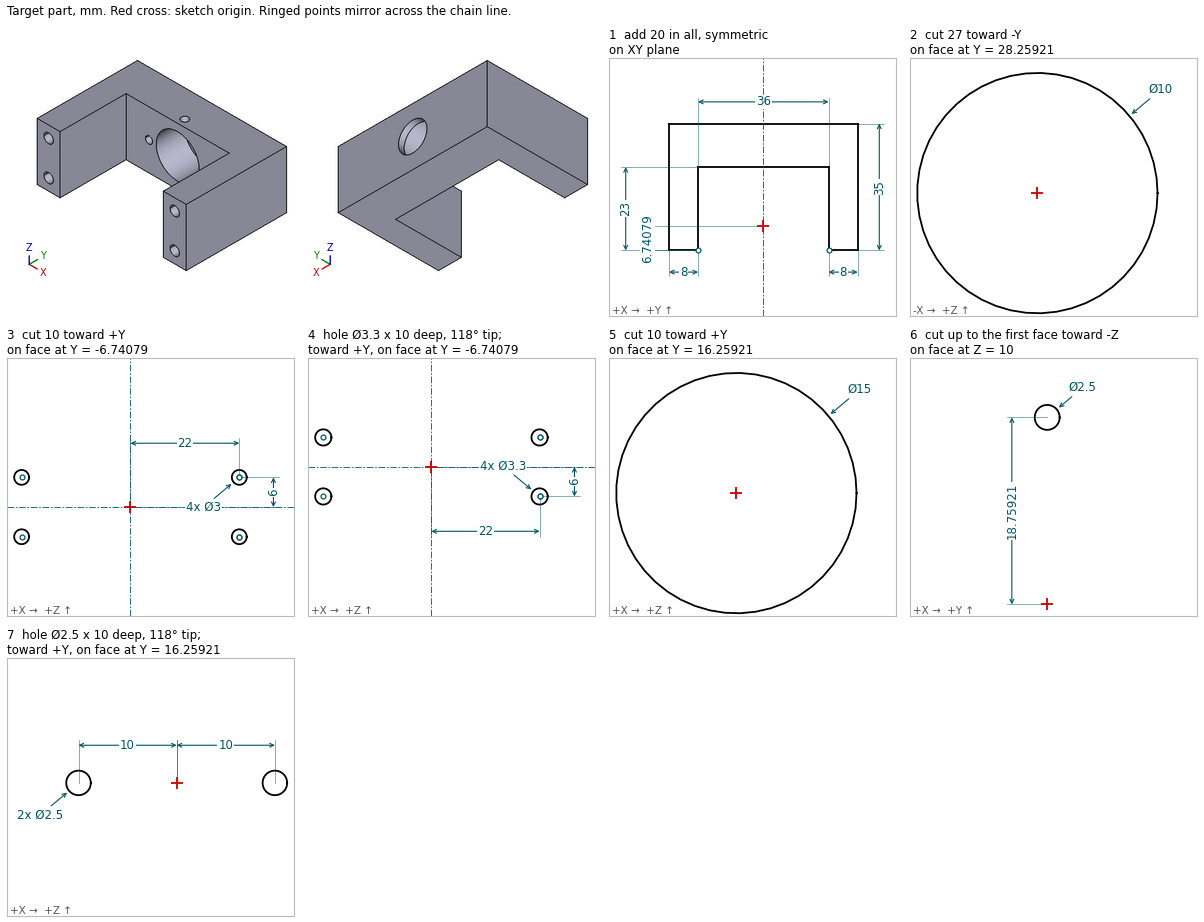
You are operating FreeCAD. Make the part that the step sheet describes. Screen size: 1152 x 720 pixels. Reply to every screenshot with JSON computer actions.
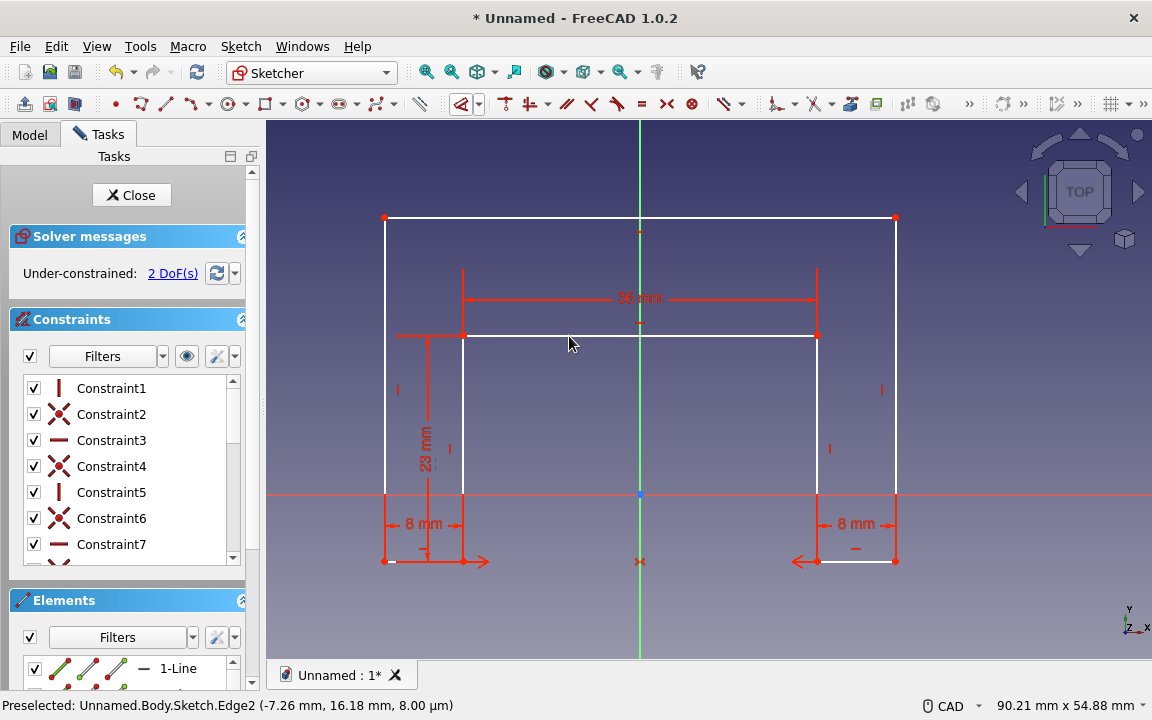
{"action": "left_click", "coordinate": [896, 459]}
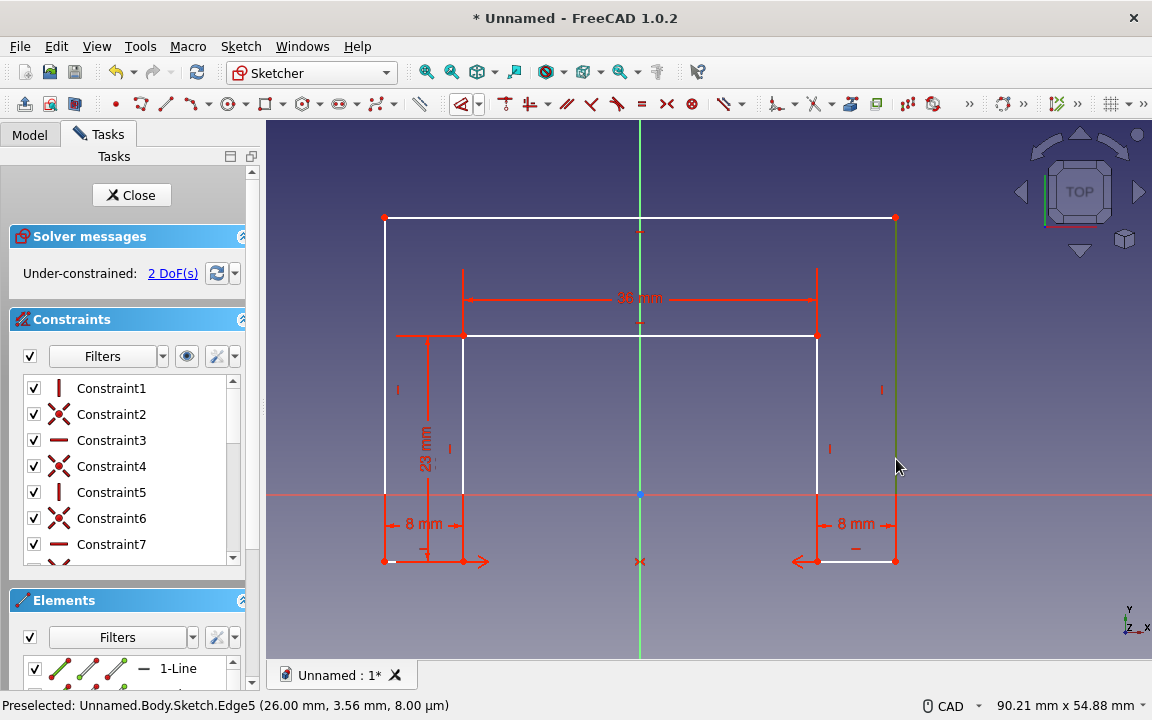
{"action": "key", "text": "i"}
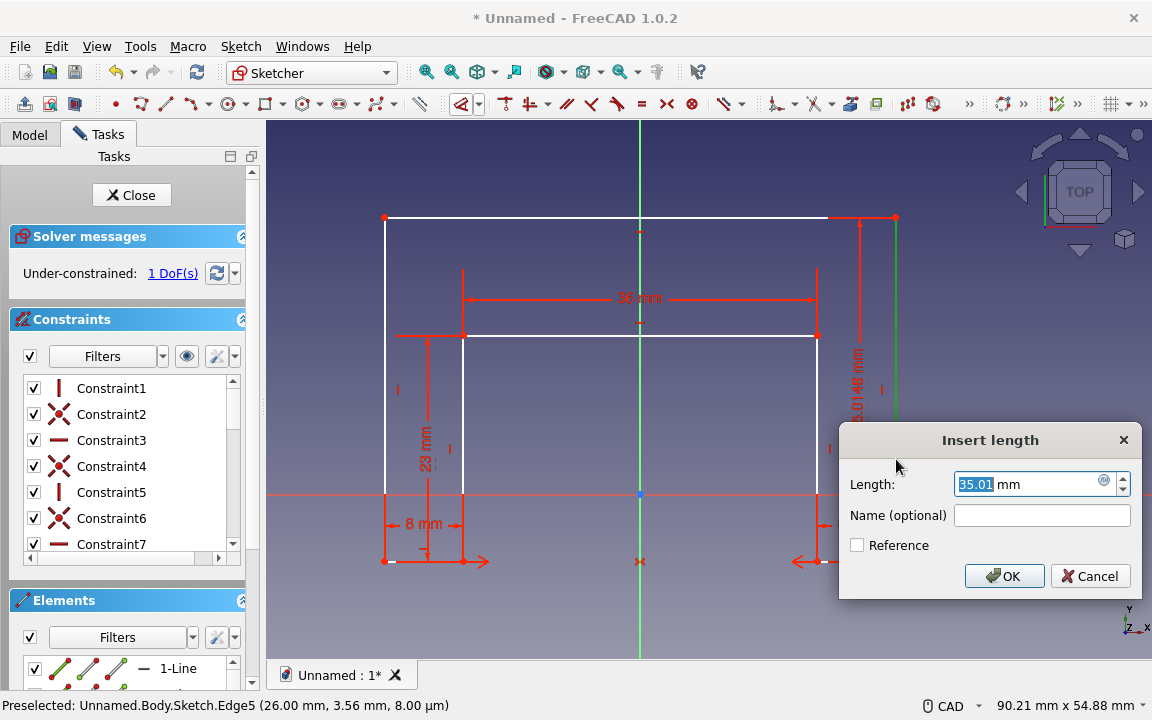
{"action": "type", "text": "35"}
{"action": "key", "text": "Return"}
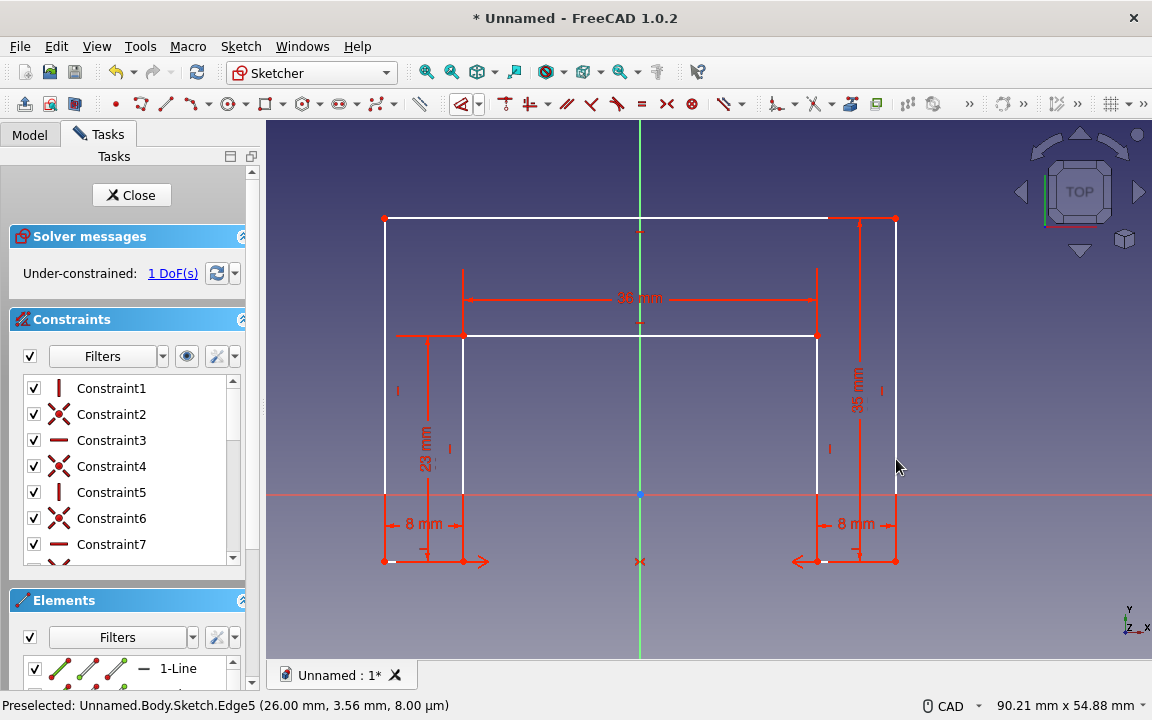
{"action": "left_click", "coordinate": [463, 562]}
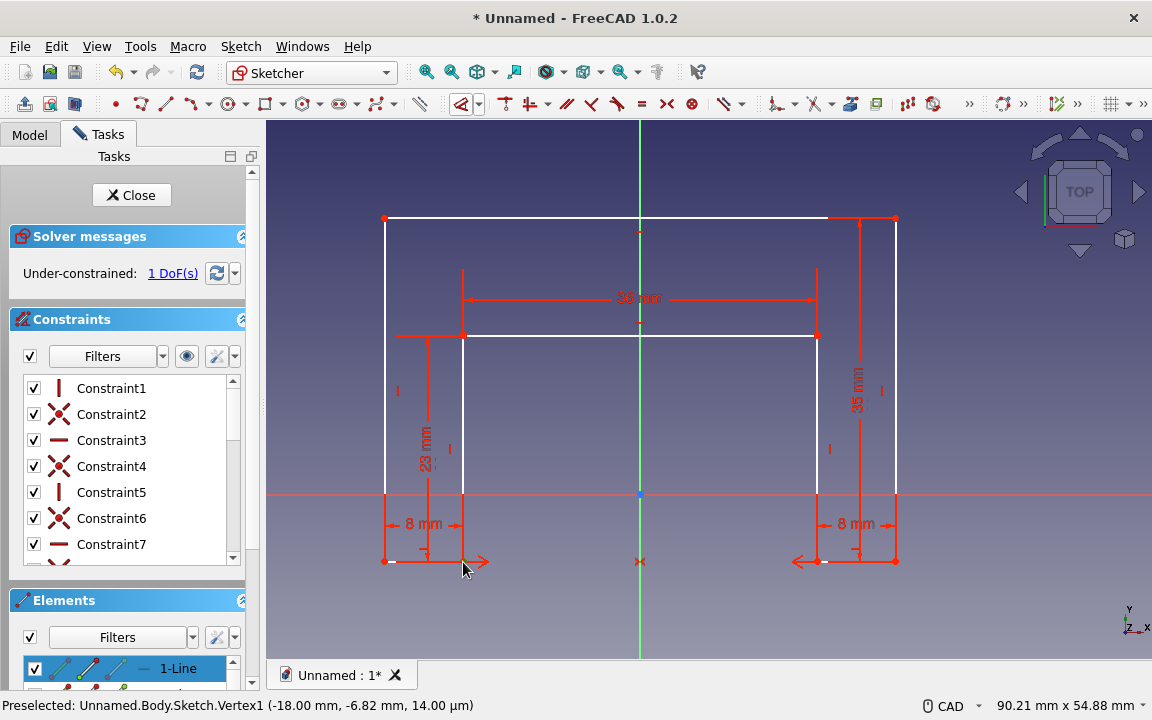
{"action": "key", "text": "i"}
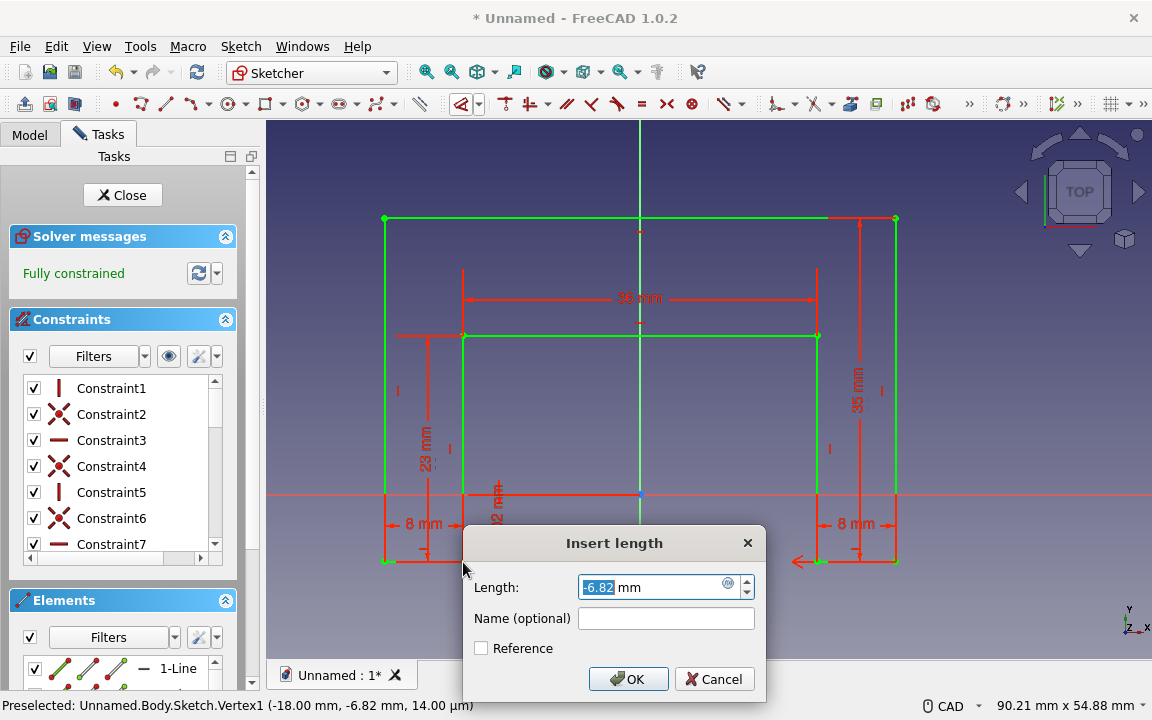
{"action": "type", "text": "-6.74079"}
{"action": "key", "text": "Return"}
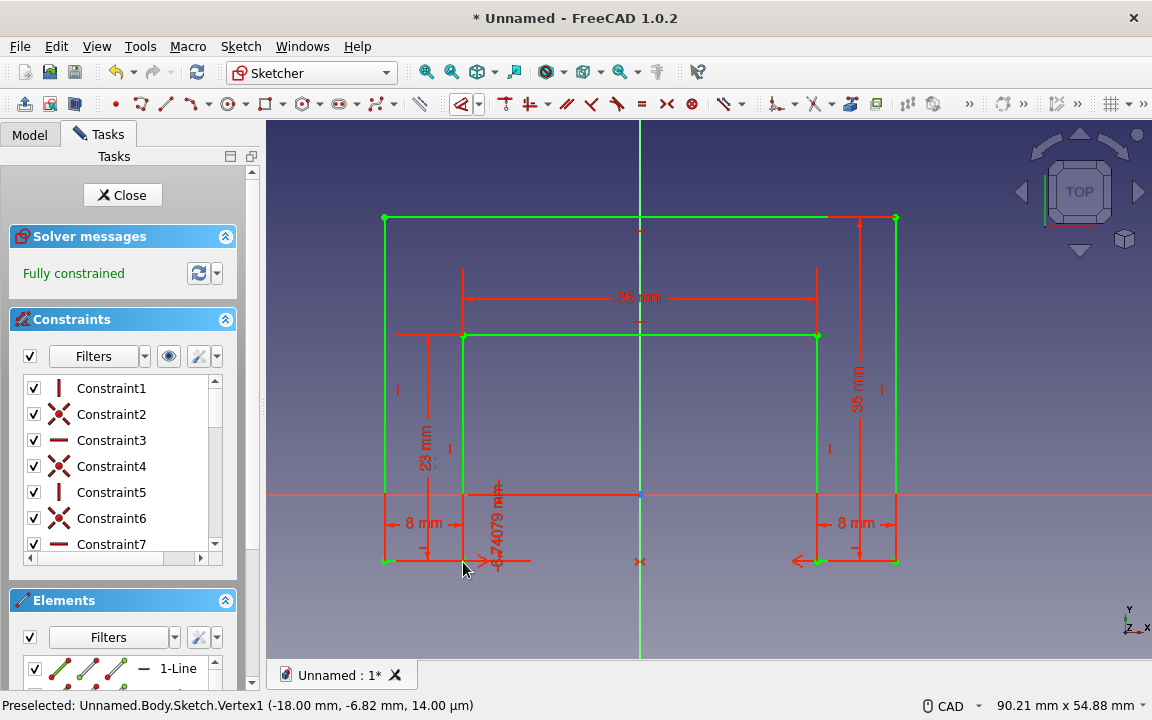
{"action": "left_click", "coordinate": [123, 195]}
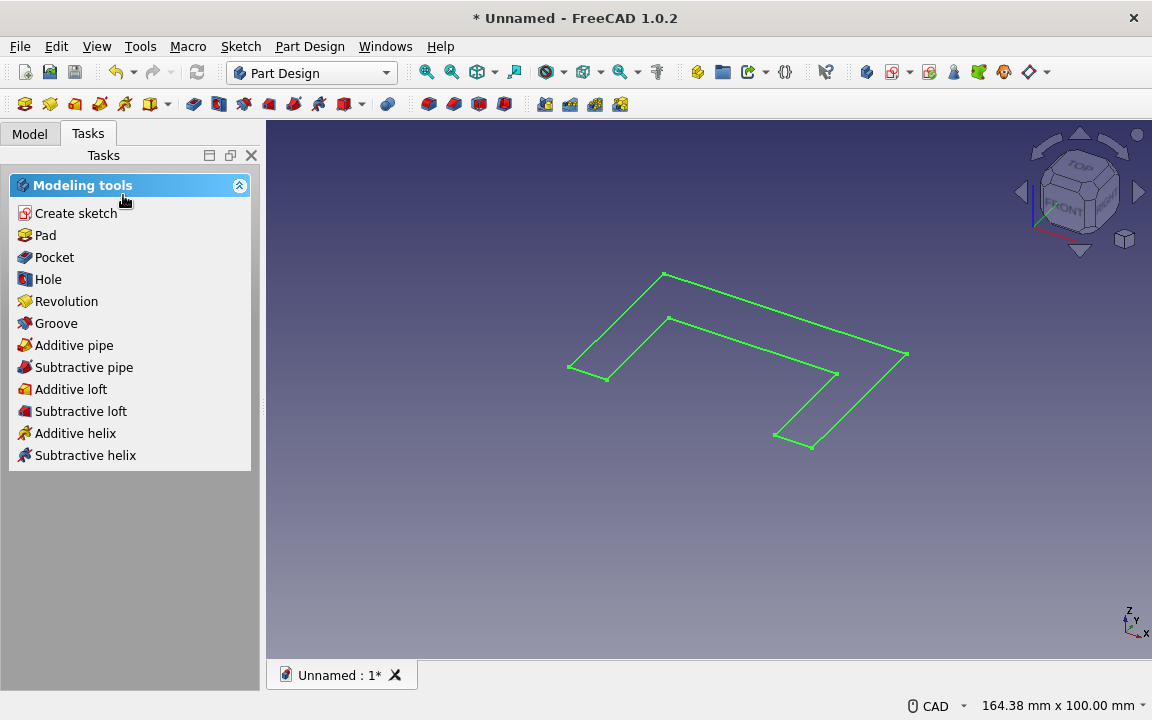
{"action": "left_click", "coordinate": [25, 104]}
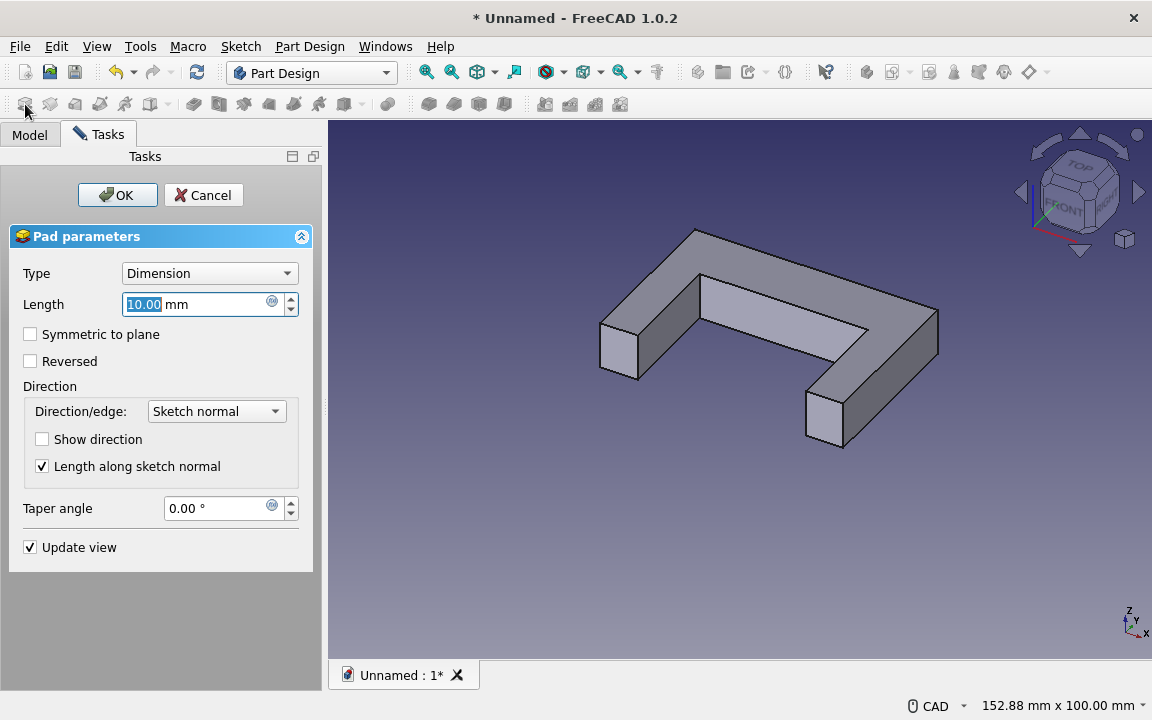
{"action": "type", "text": "20"}
{"action": "key", "text": "Tab"}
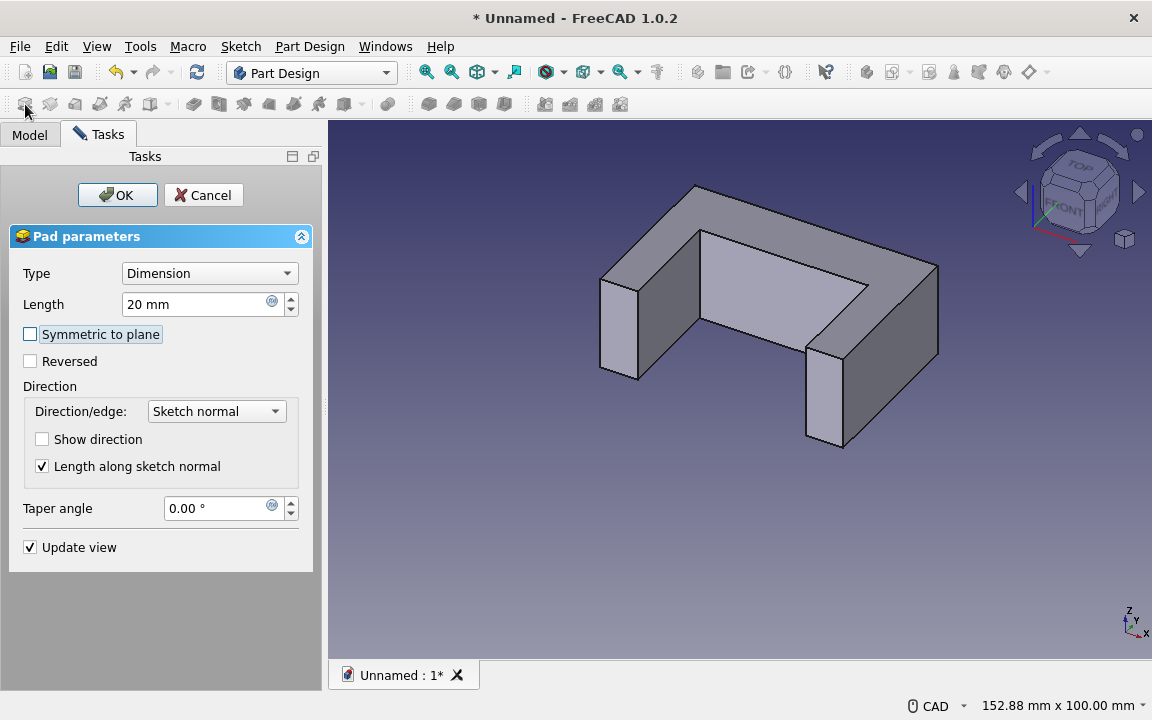
{"action": "left_click", "coordinate": [31, 334]}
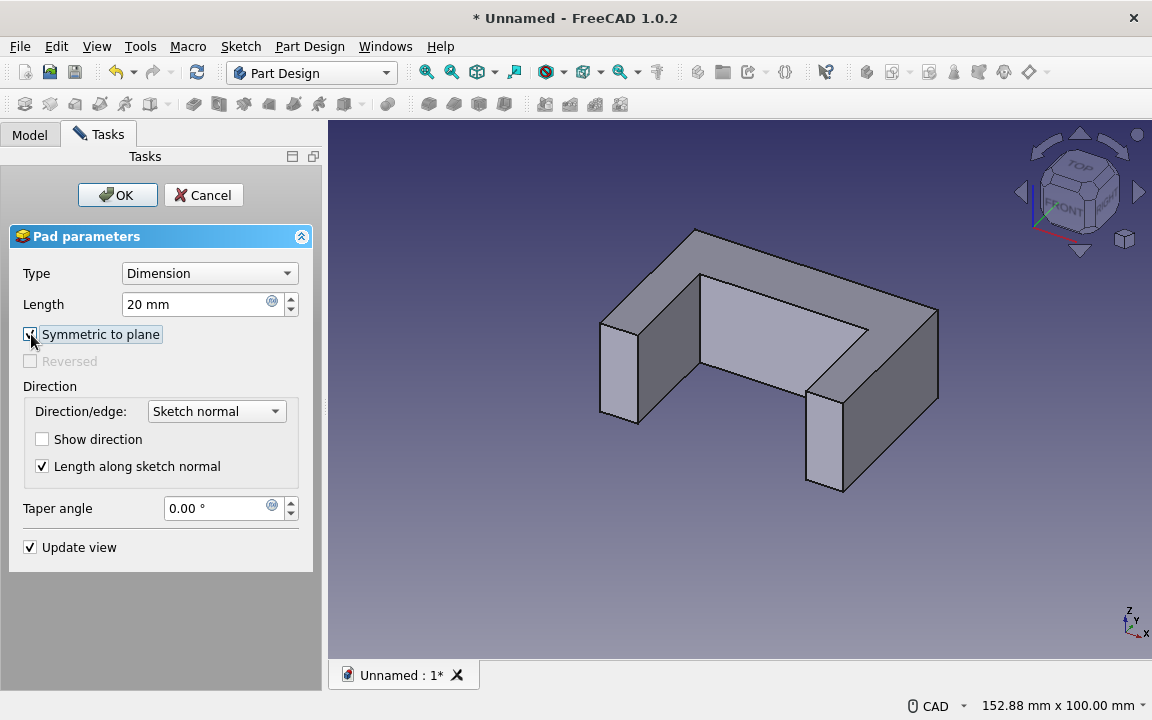
{"action": "left_click", "coordinate": [118, 195]}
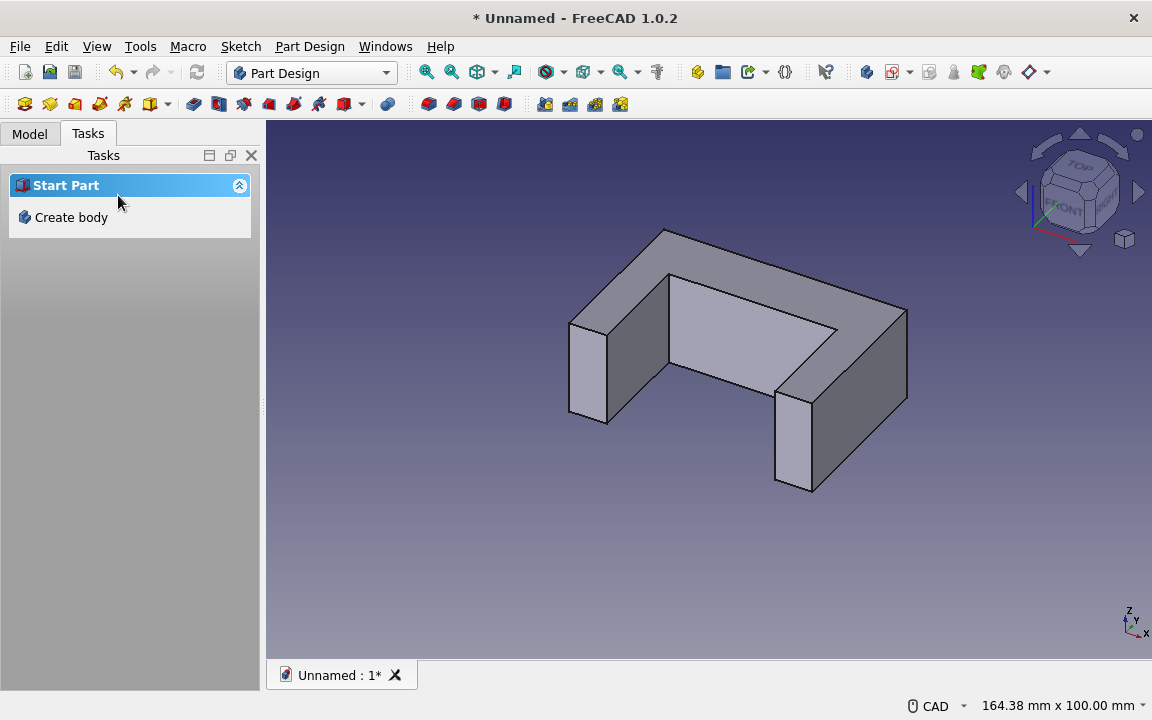
{"action": "key", "text": "4"}